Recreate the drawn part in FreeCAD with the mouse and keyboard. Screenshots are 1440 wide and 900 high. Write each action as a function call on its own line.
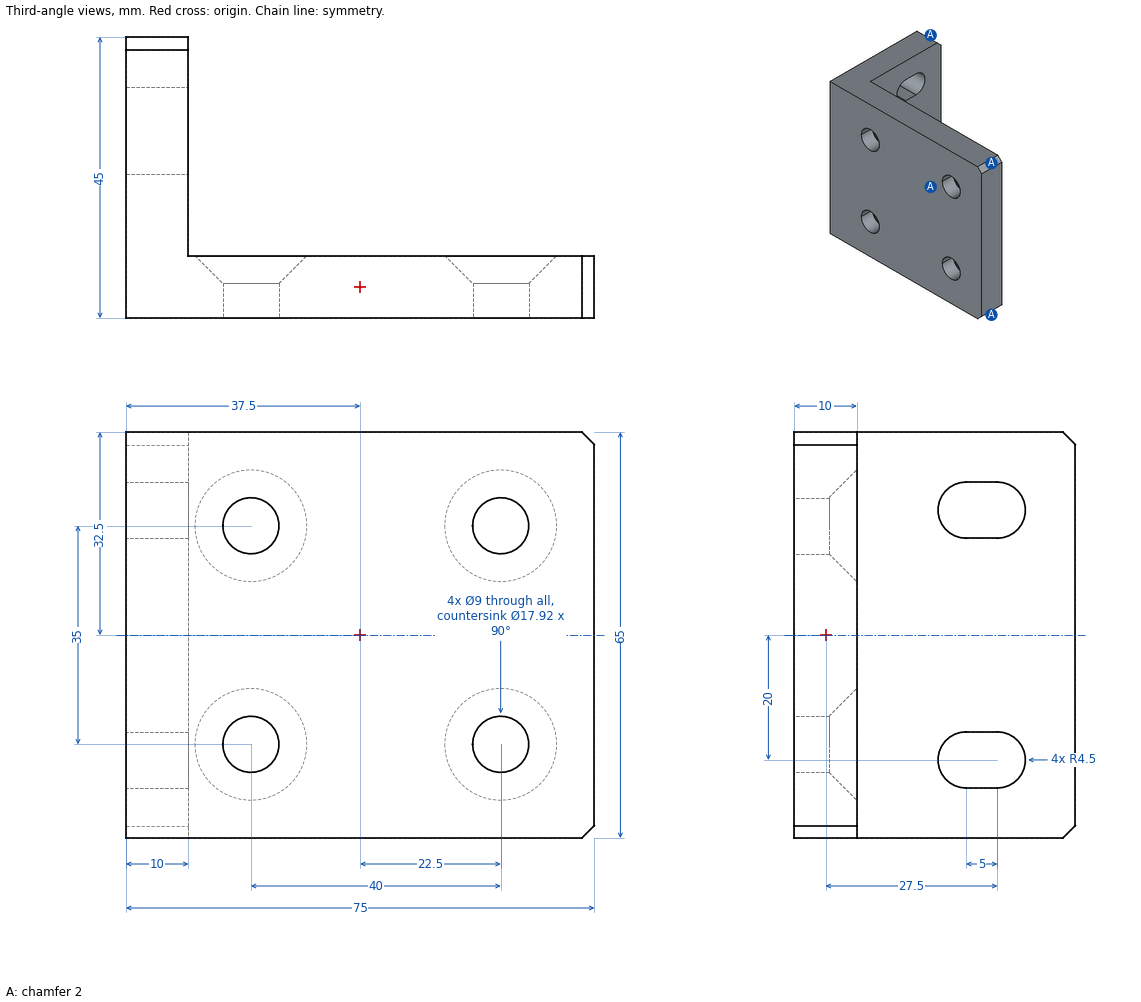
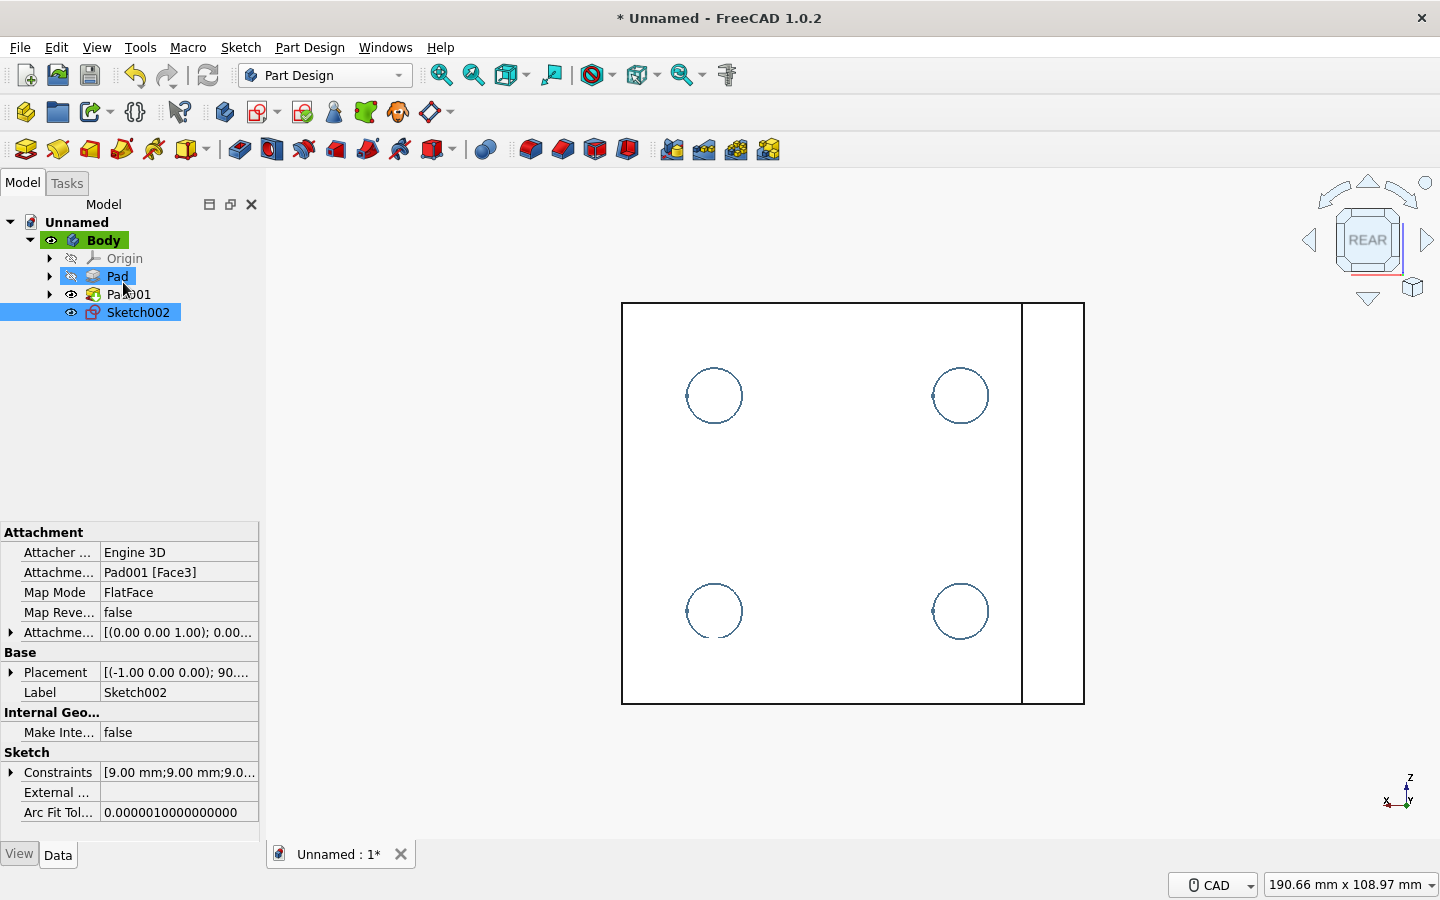
click(272, 150)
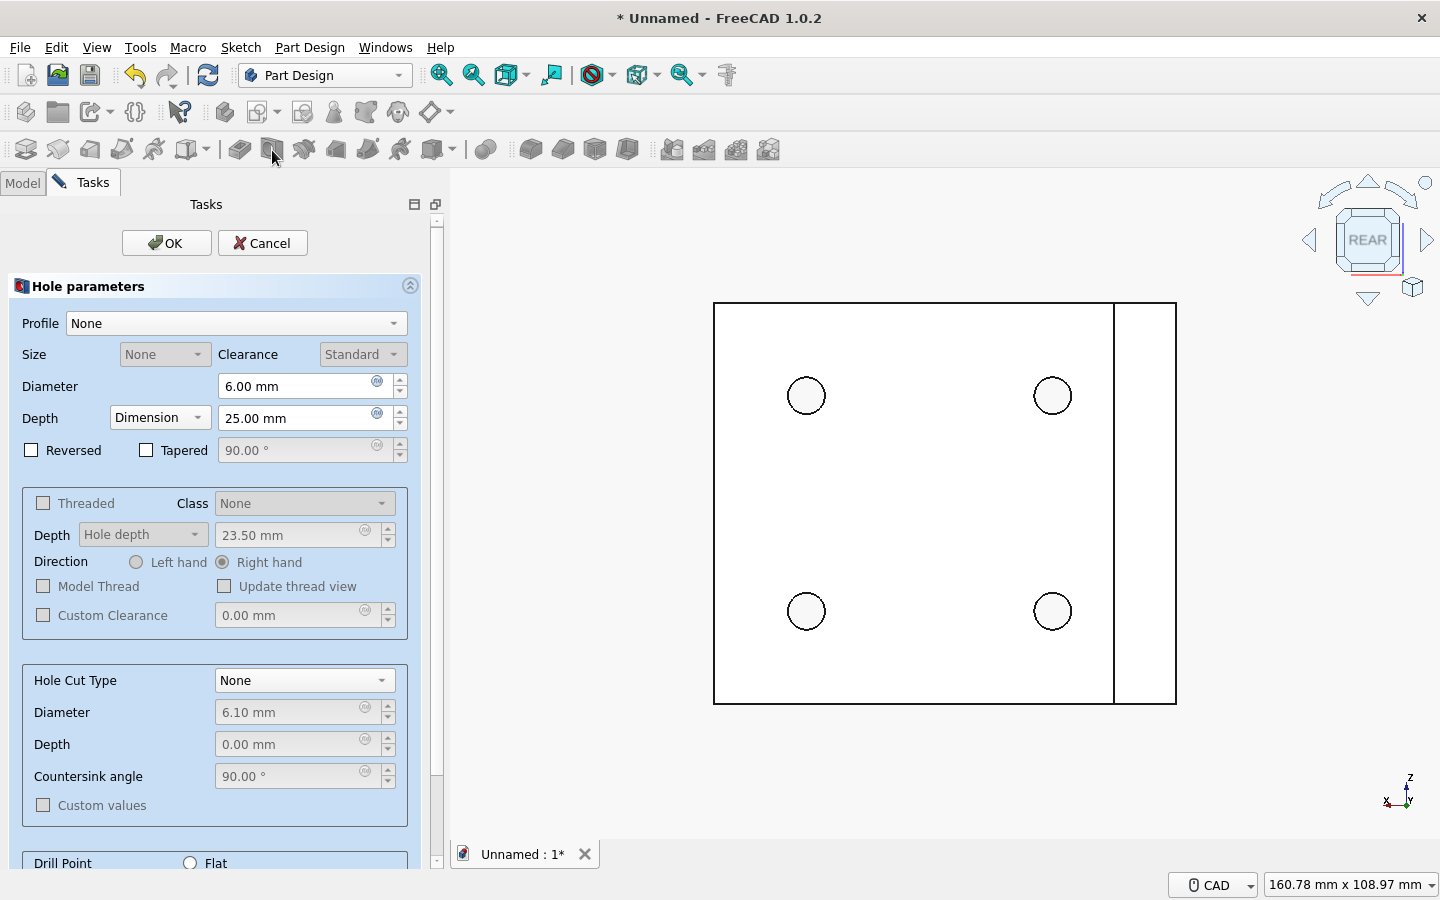
triple_click(305, 386)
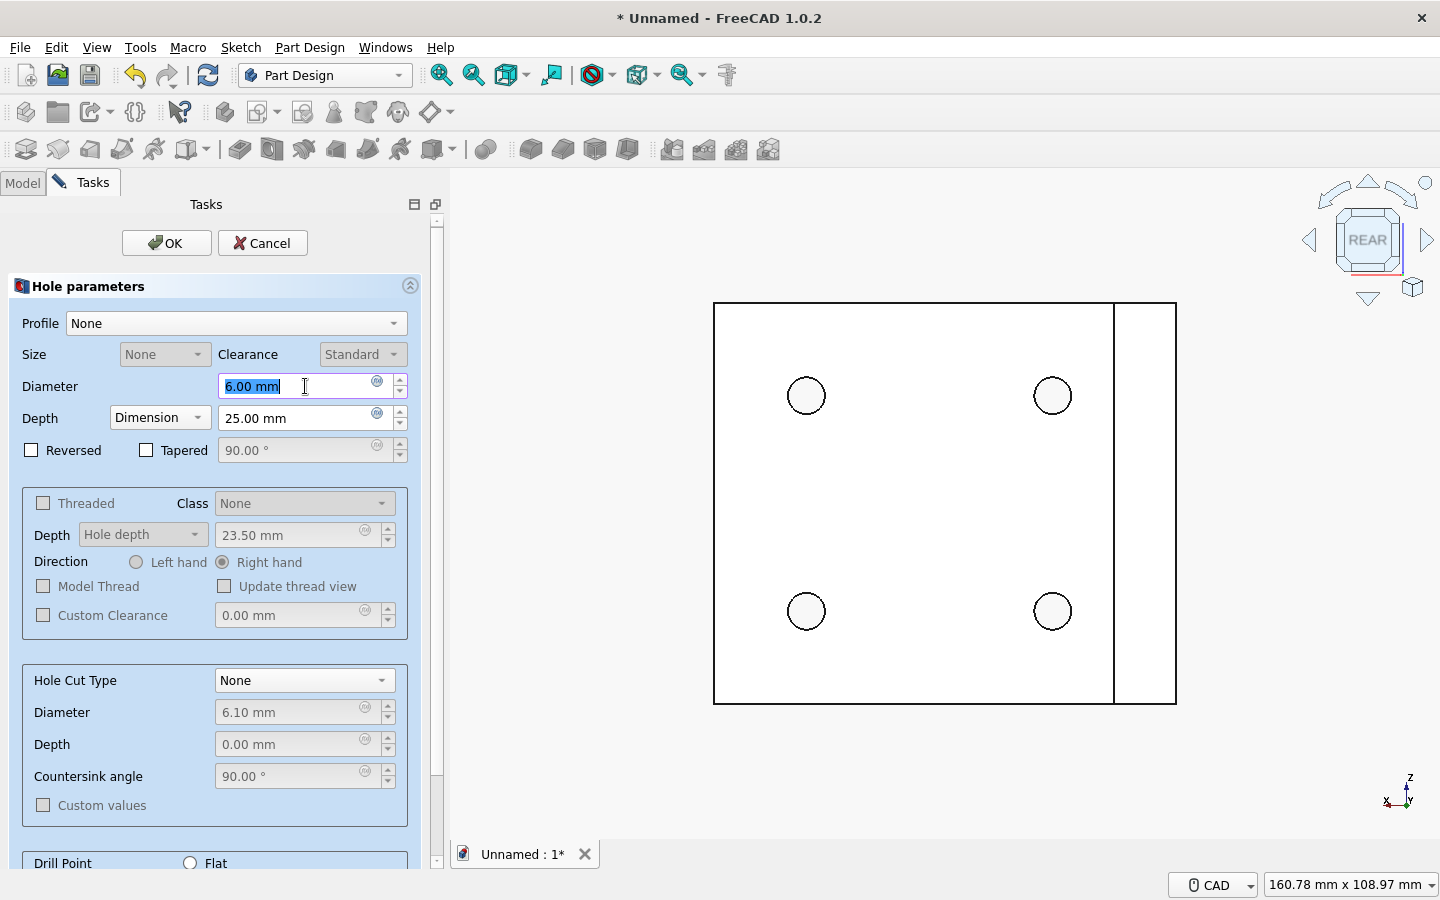
text(9)
key(Tab)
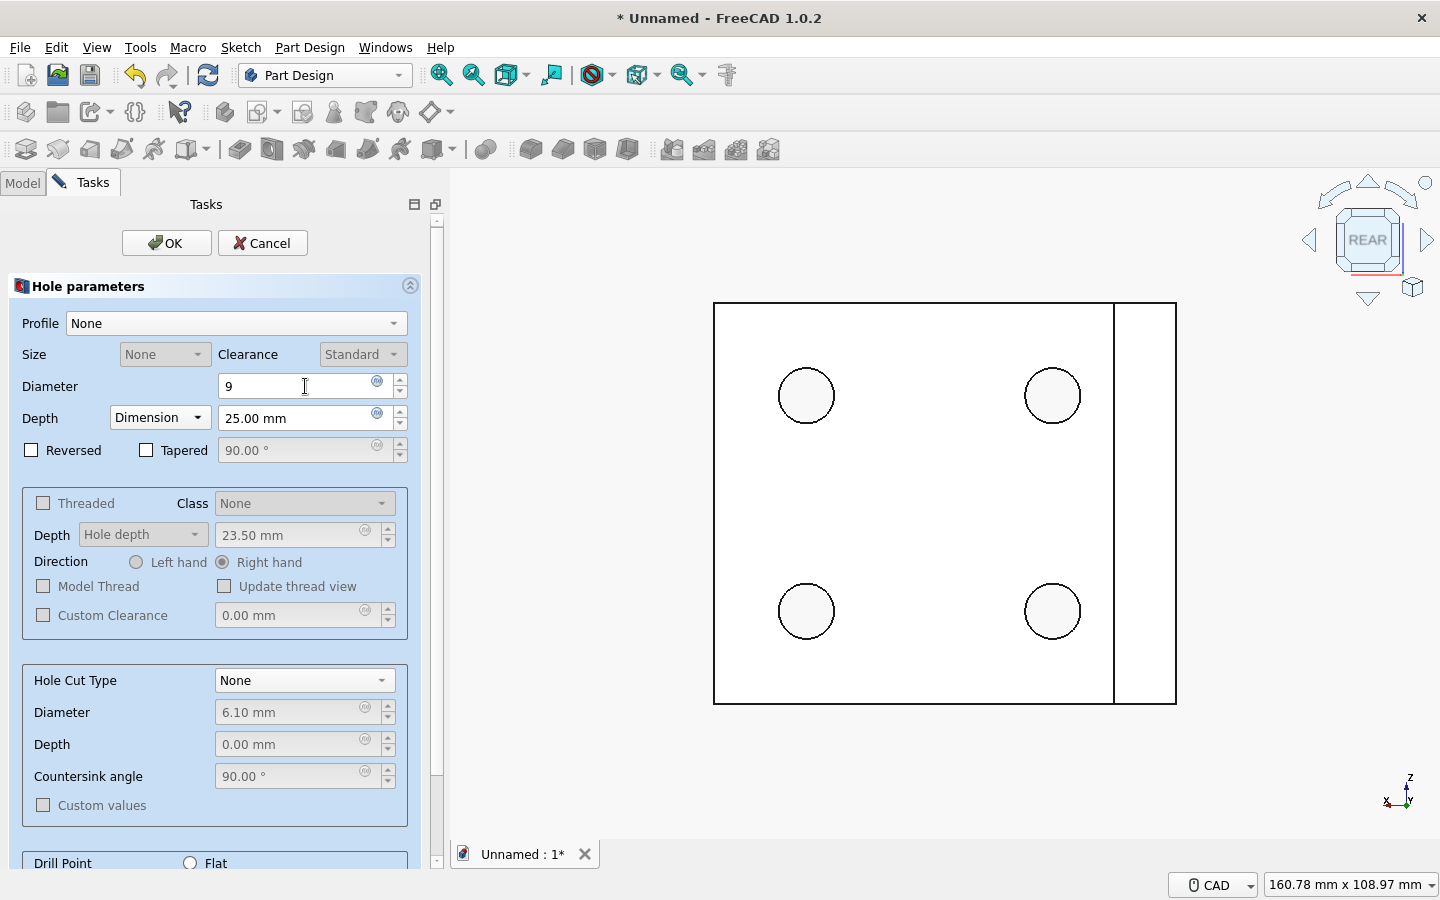
click(161, 418)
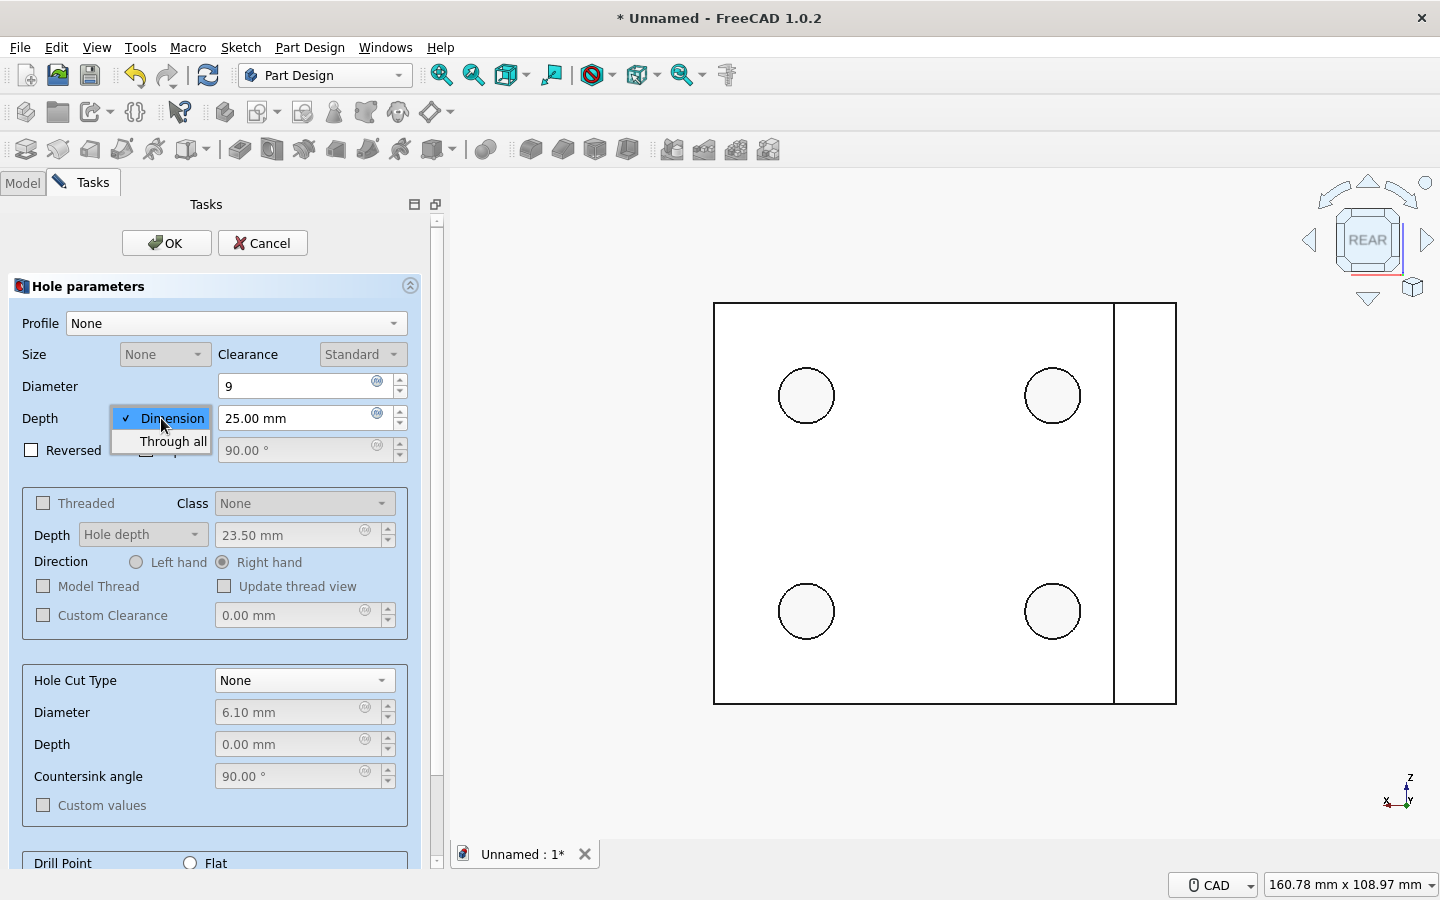
click(160, 442)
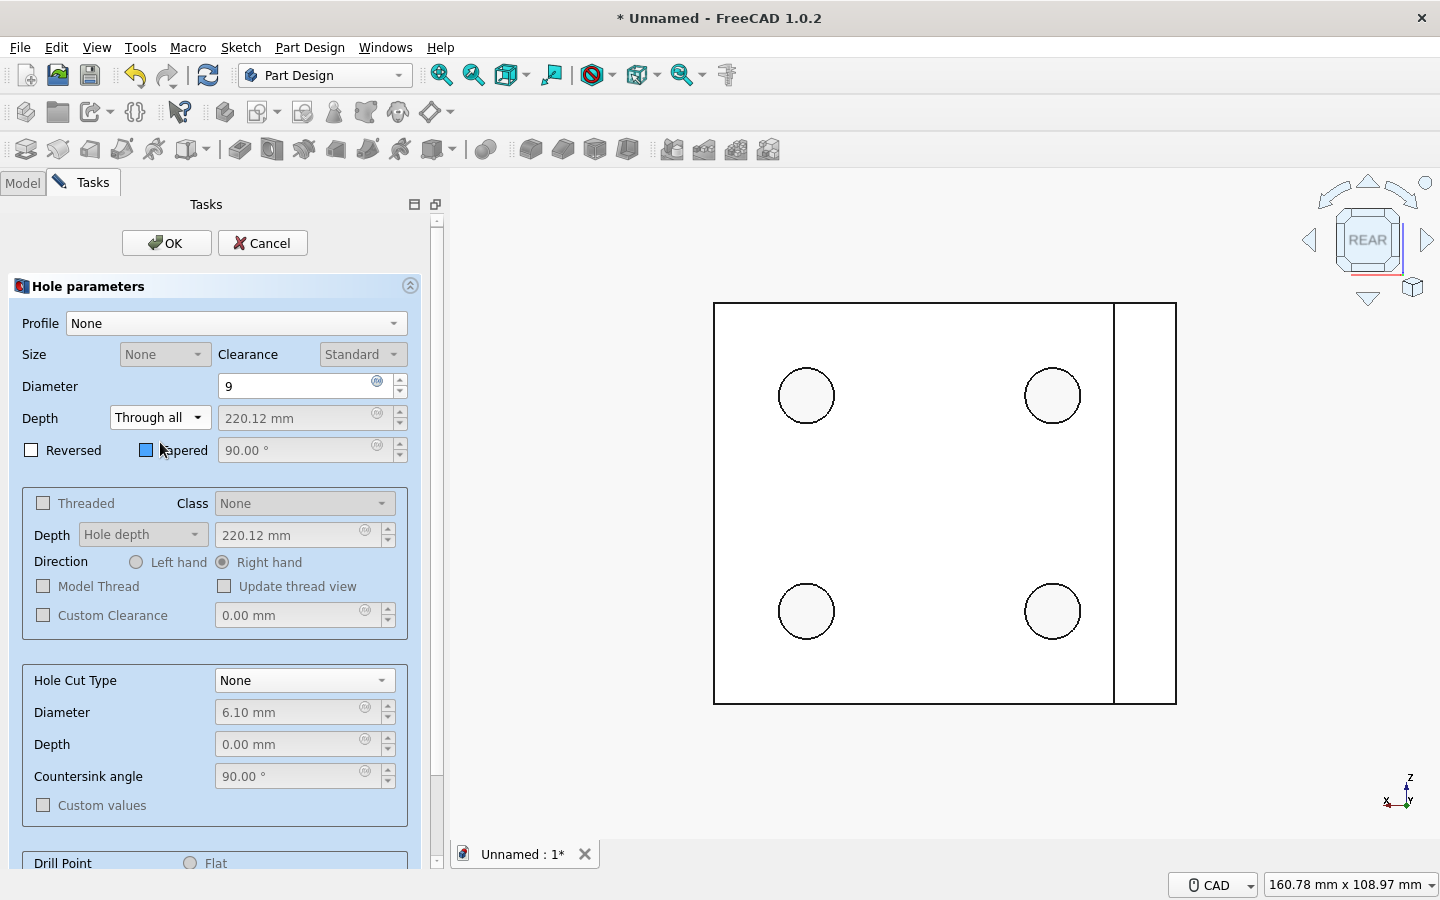
click(306, 680)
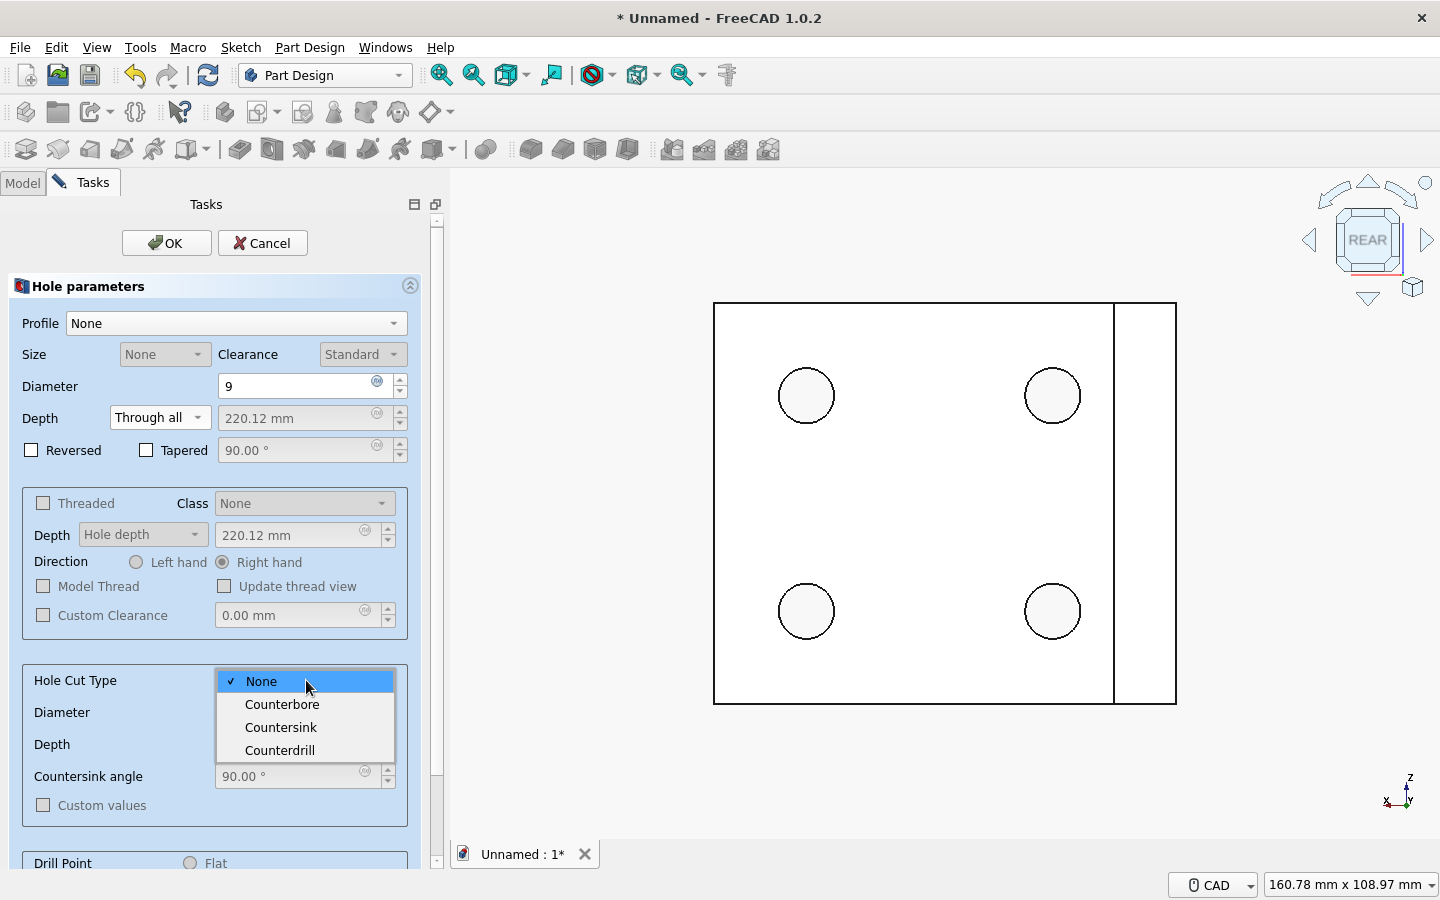
click(304, 728)